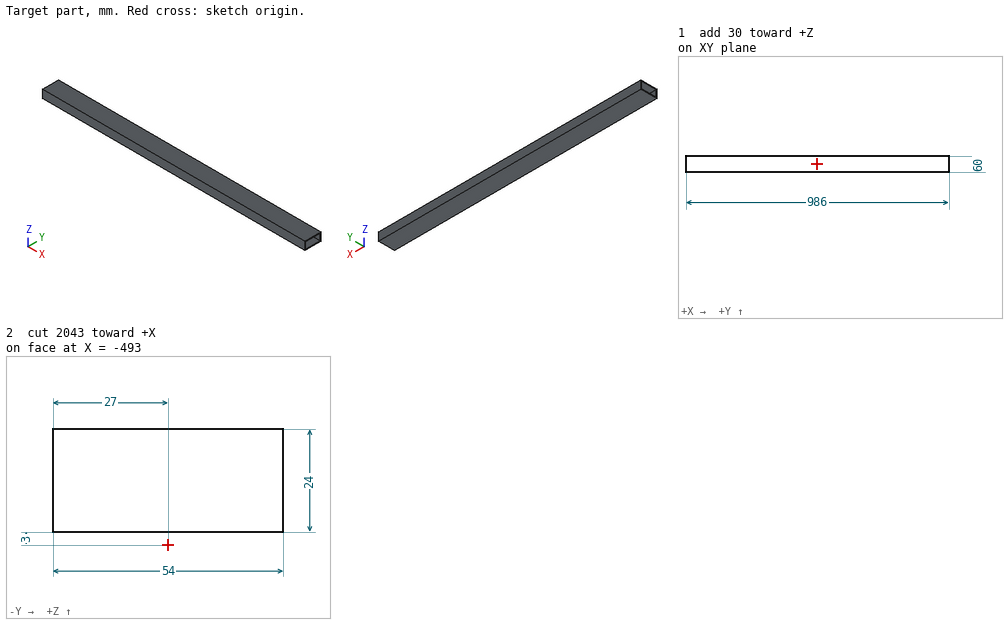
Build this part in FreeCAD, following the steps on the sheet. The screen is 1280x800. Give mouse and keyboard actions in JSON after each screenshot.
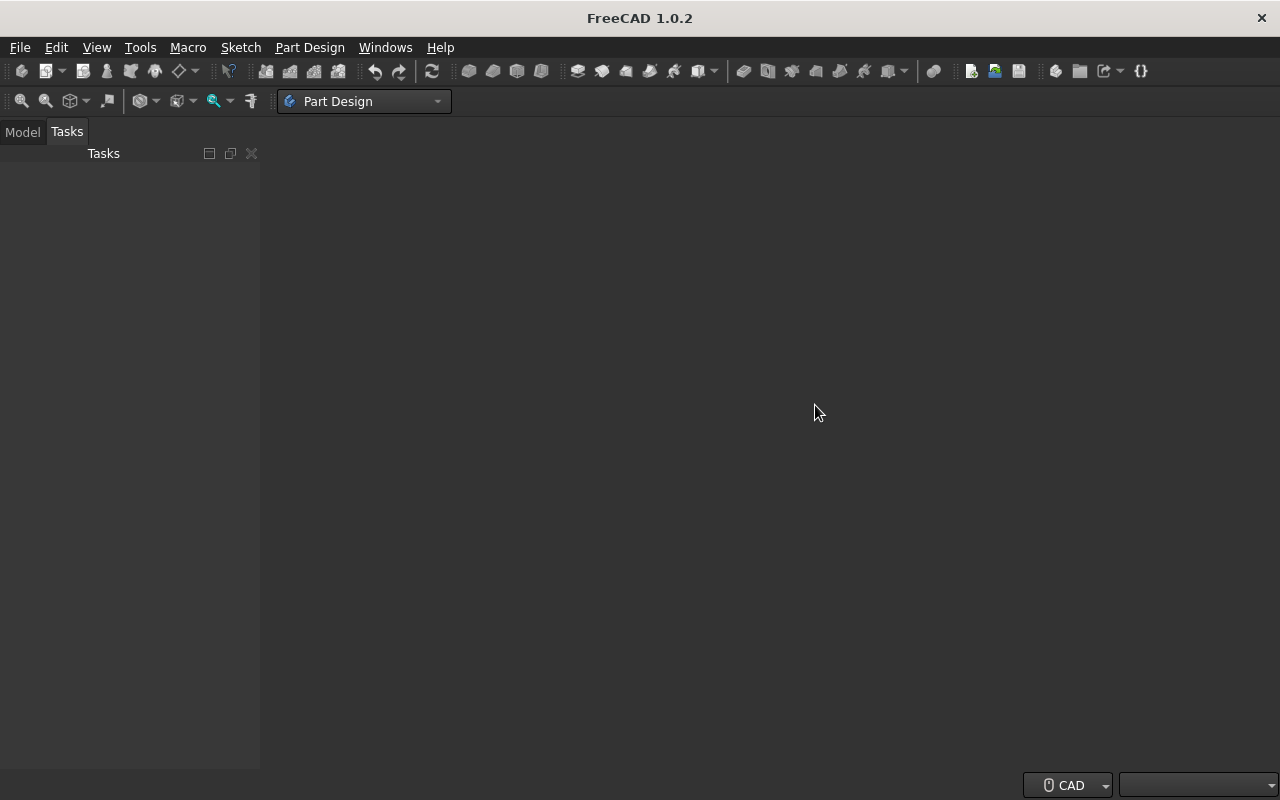
{"action": "left_click", "coordinate": [972, 72]}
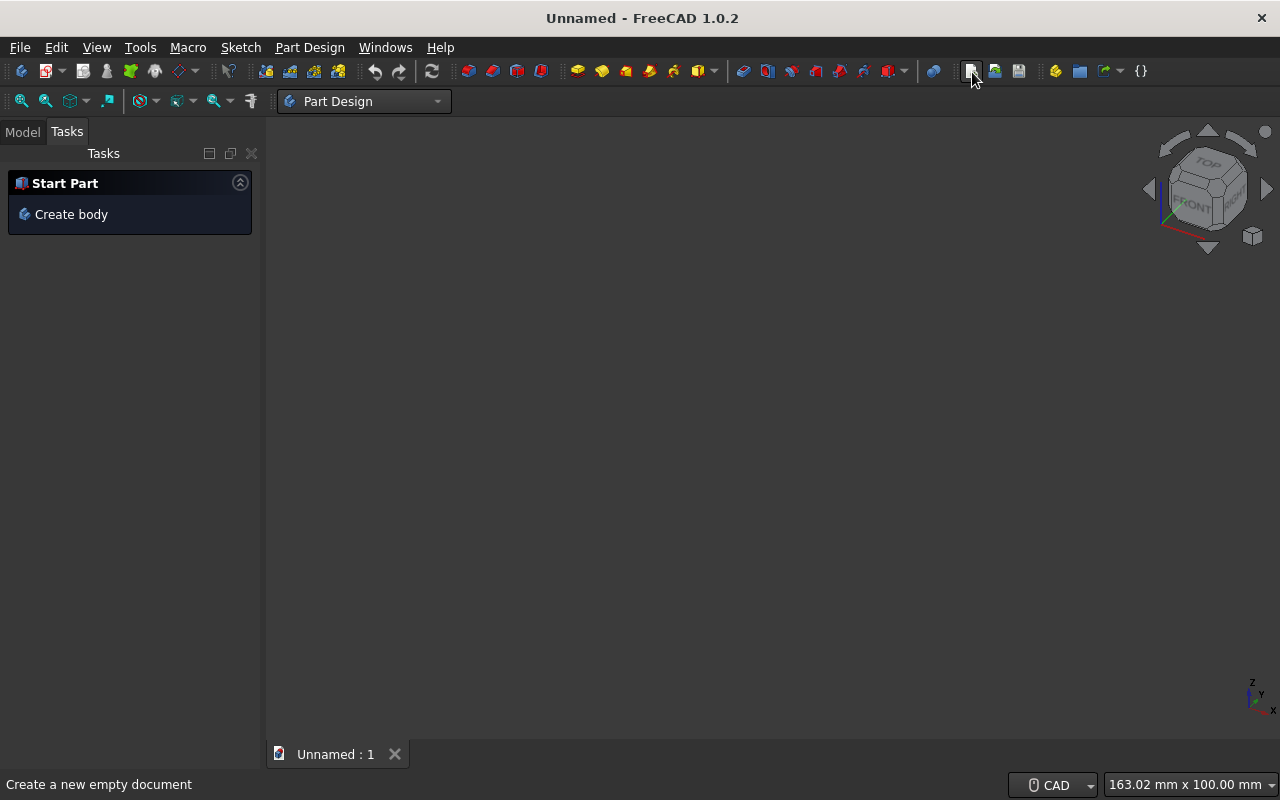
{"action": "left_click", "coordinate": [46, 72]}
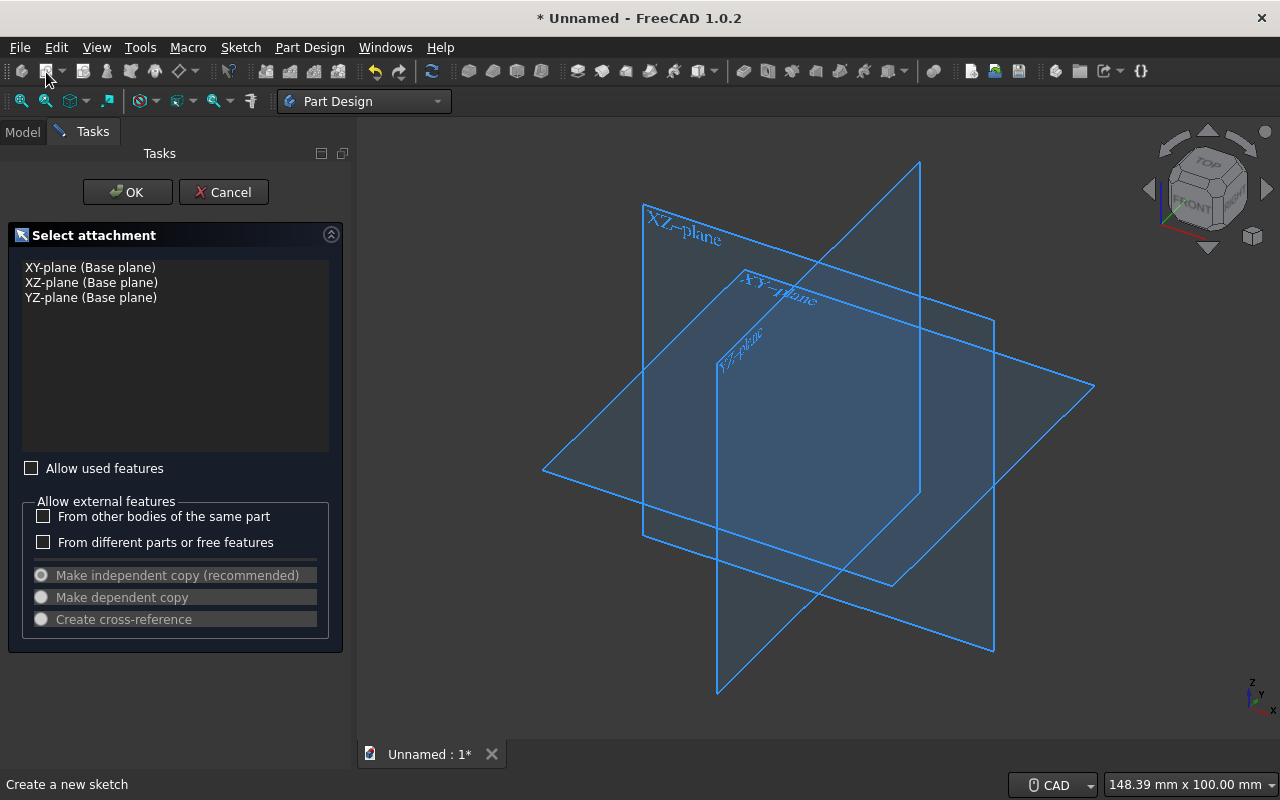
{"action": "left_click", "coordinate": [82, 268]}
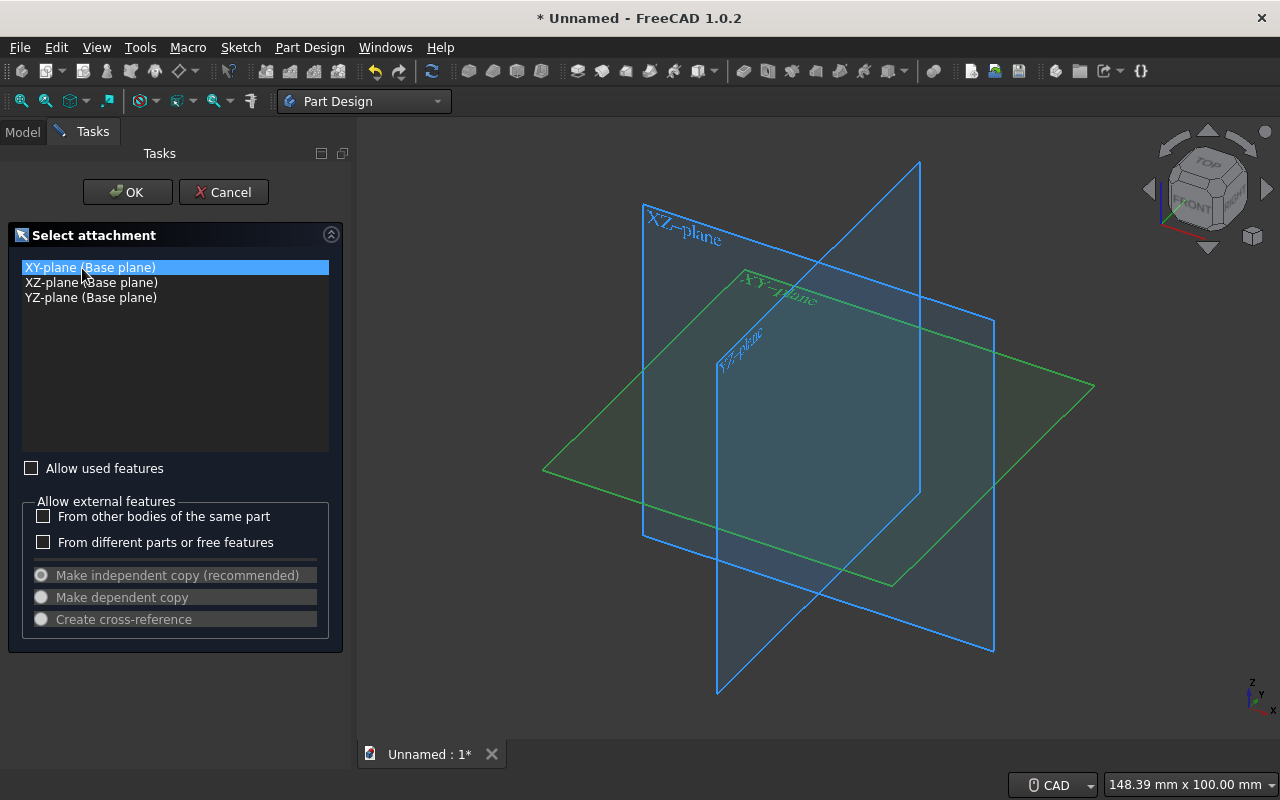
{"action": "left_click", "coordinate": [128, 192]}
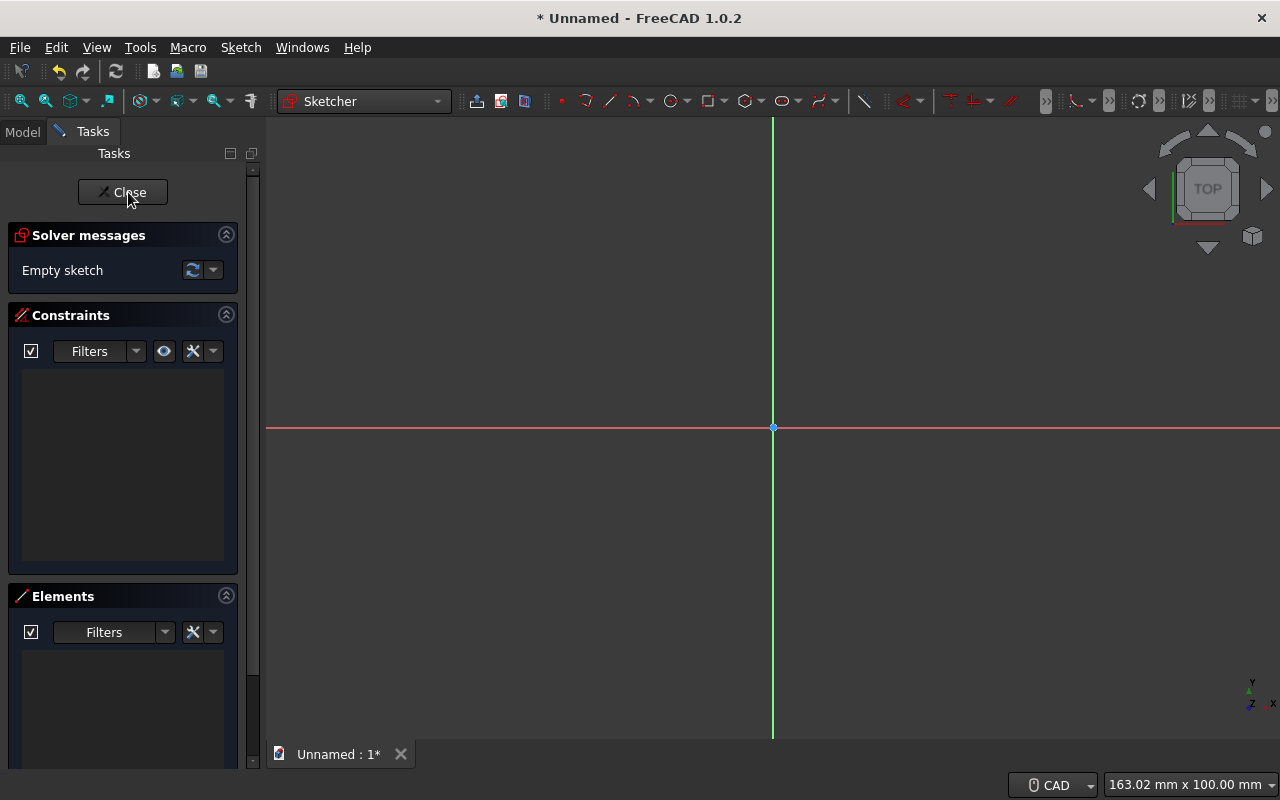
{"action": "scroll", "coordinate": [698, 428], "scroll_direction": "down", "scroll_amount": 12}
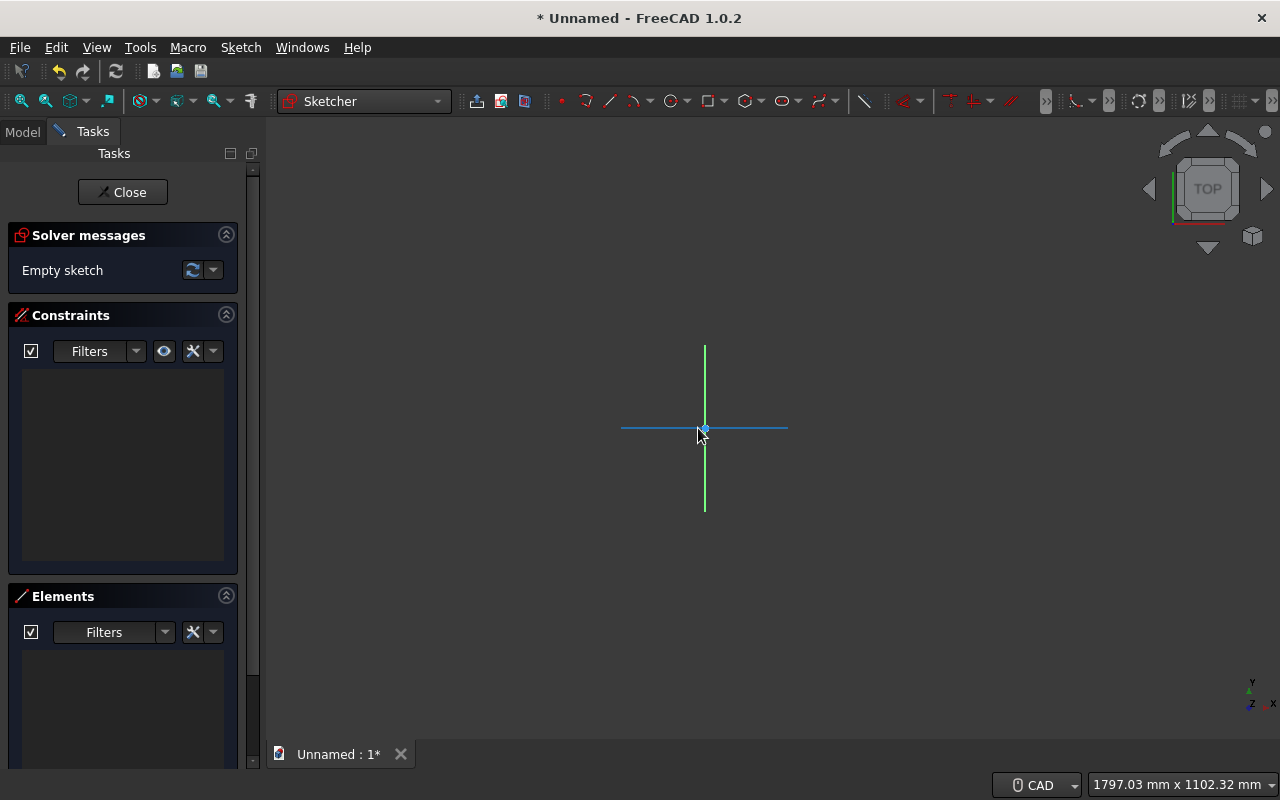
{"action": "left_click", "coordinate": [726, 102]}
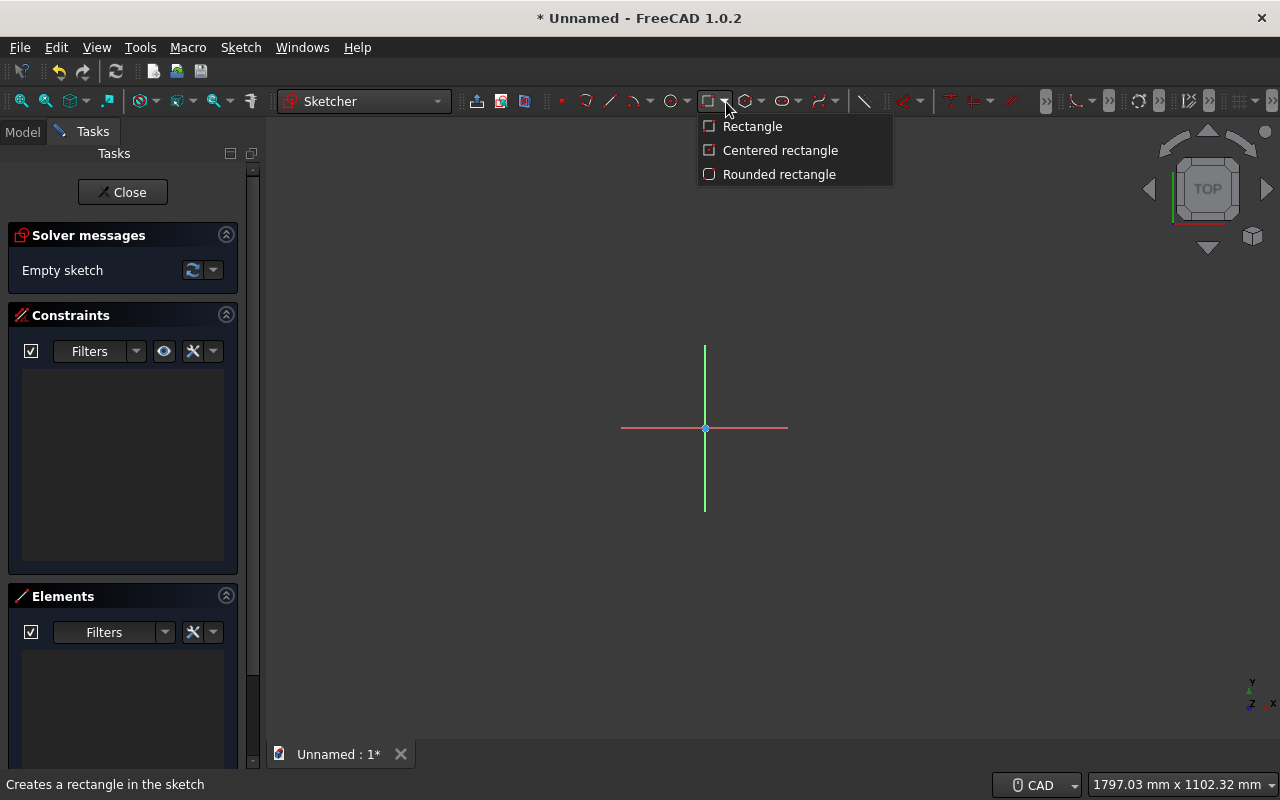
{"action": "left_click", "coordinate": [796, 150]}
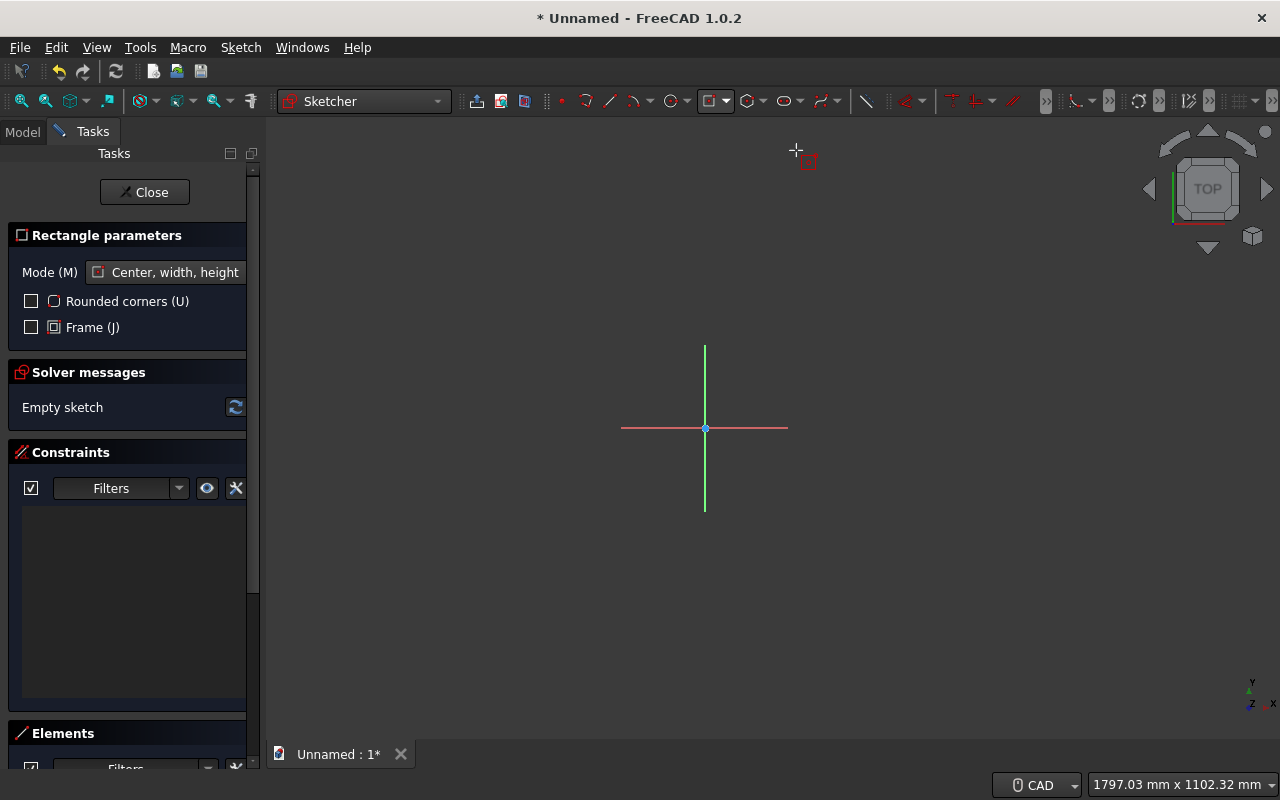
{"action": "left_click", "coordinate": [705, 428]}
{"action": "mouse_move", "coordinate": [983, 412]}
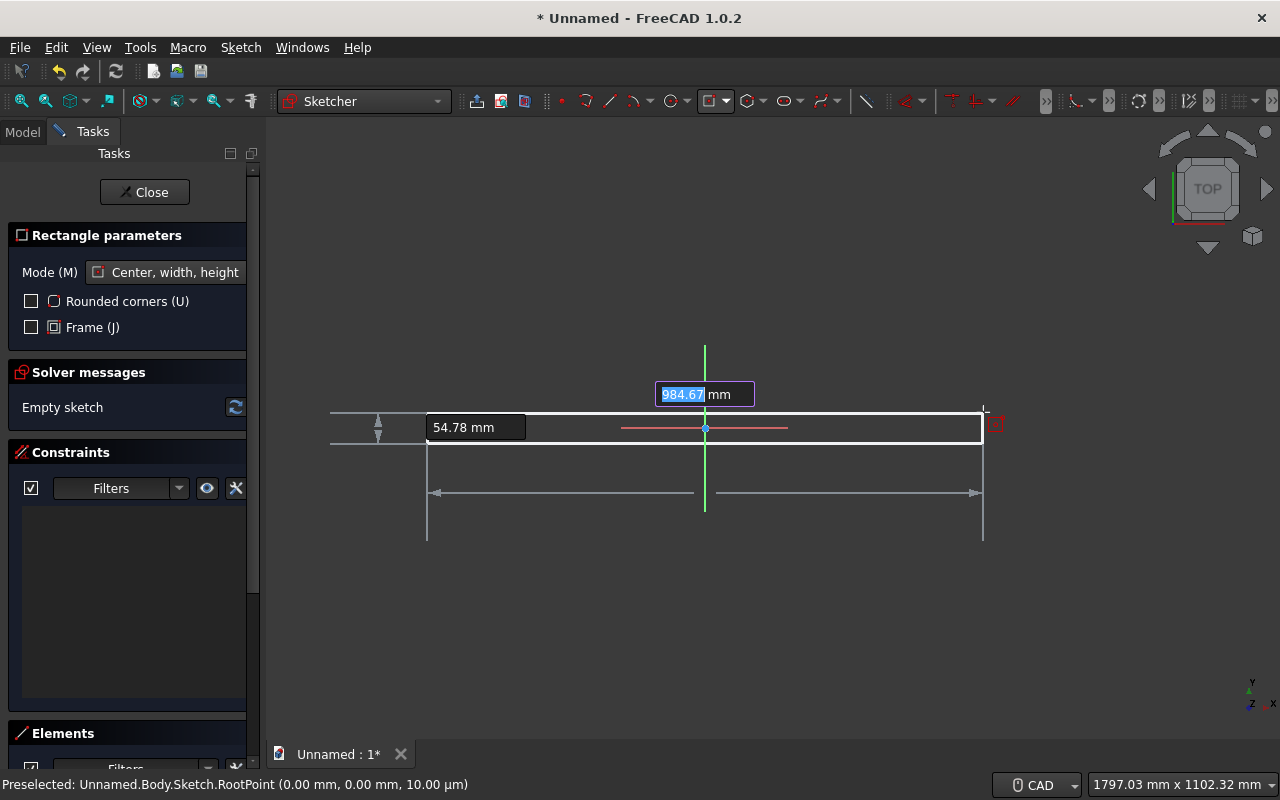
{"action": "type", "text": "986"}
{"action": "key", "text": "Tab"}
{"action": "type", "text": "60"}
{"action": "key", "text": "Return"}
{"action": "key", "text": "Escape"}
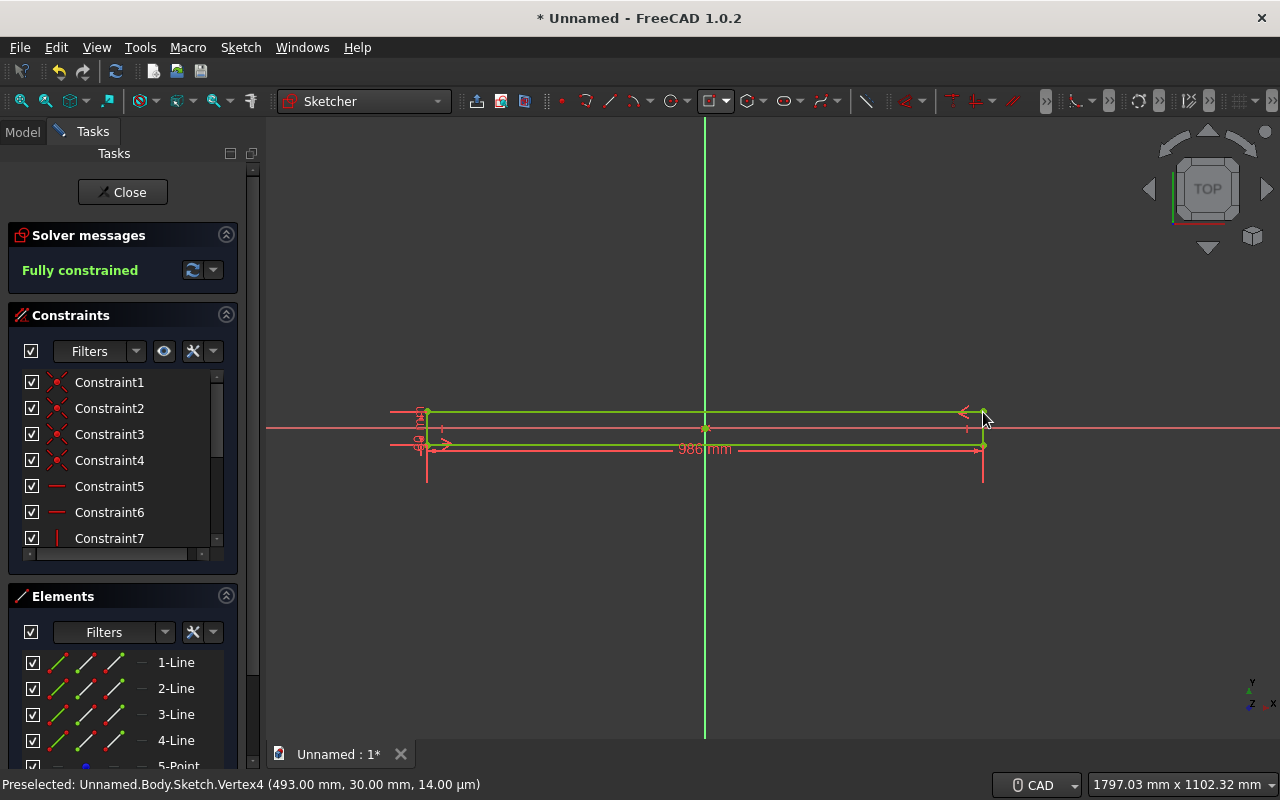
{"action": "left_click", "coordinate": [123, 192]}